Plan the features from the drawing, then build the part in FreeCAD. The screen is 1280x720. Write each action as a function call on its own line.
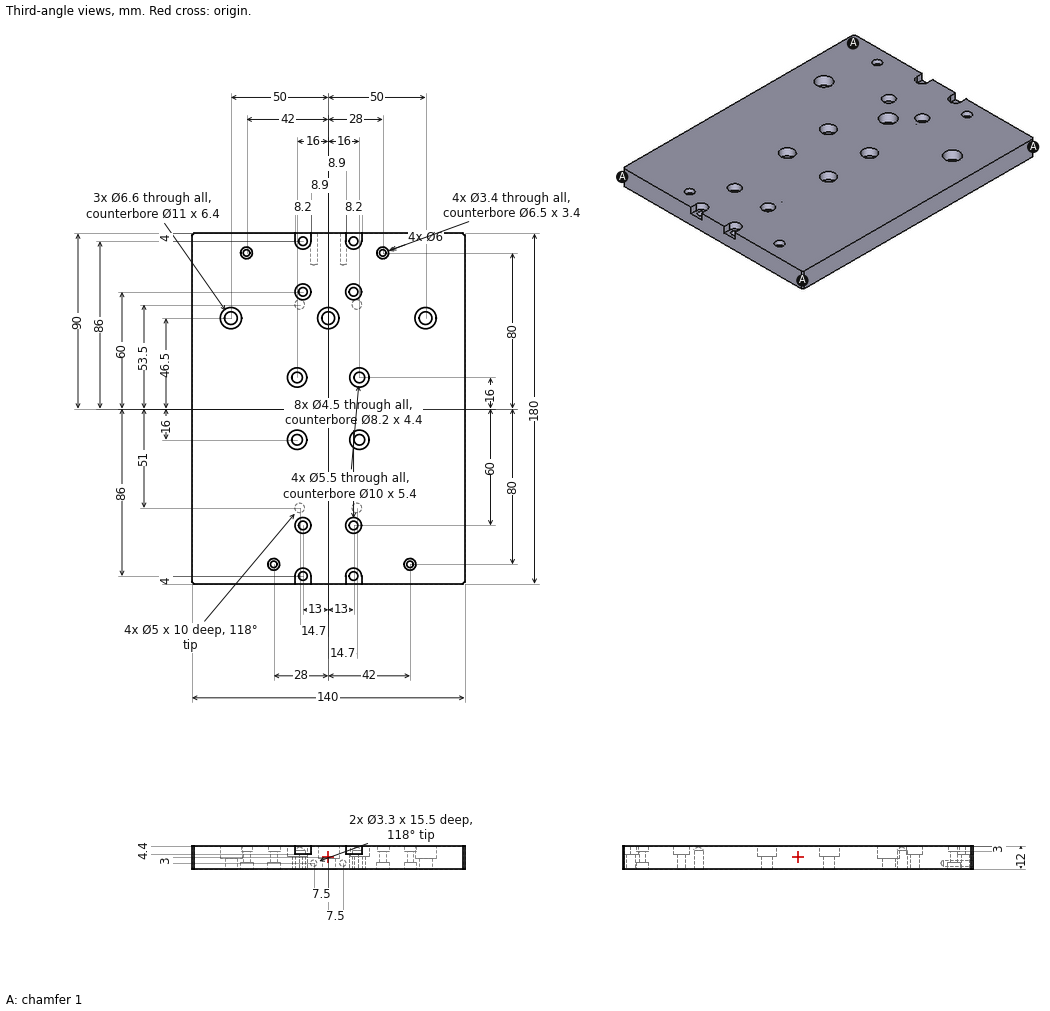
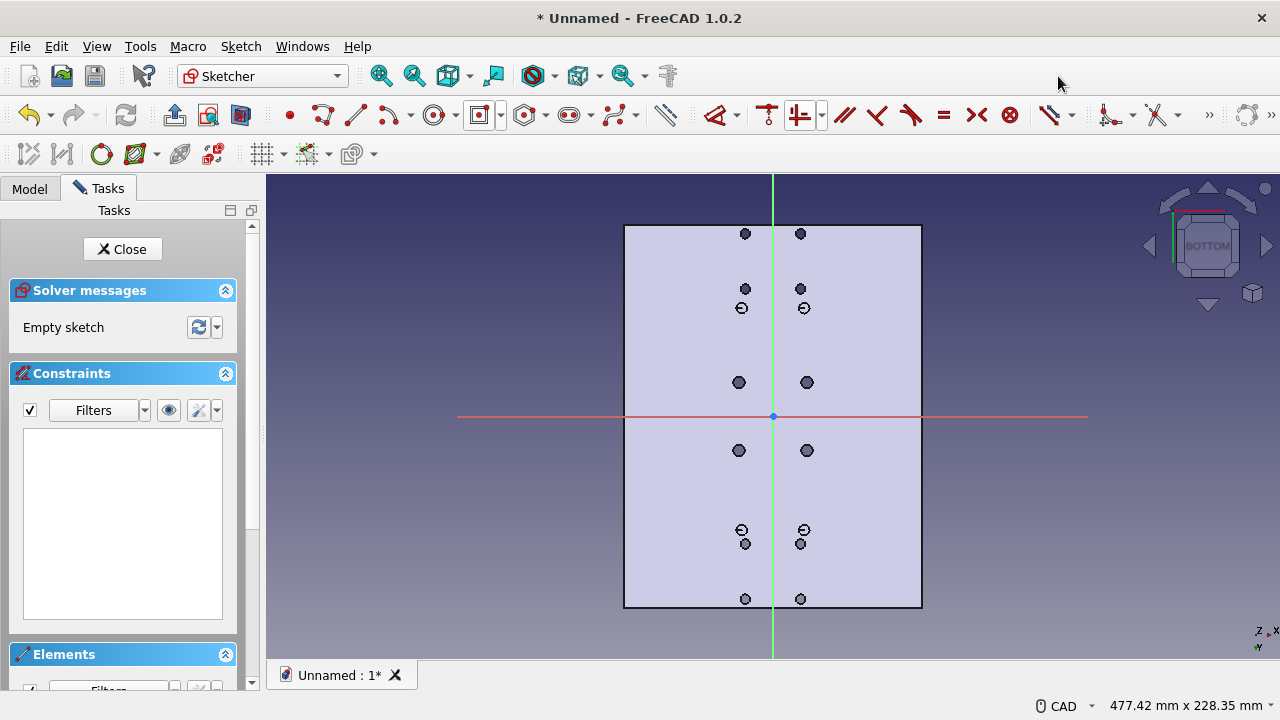
click(434, 116)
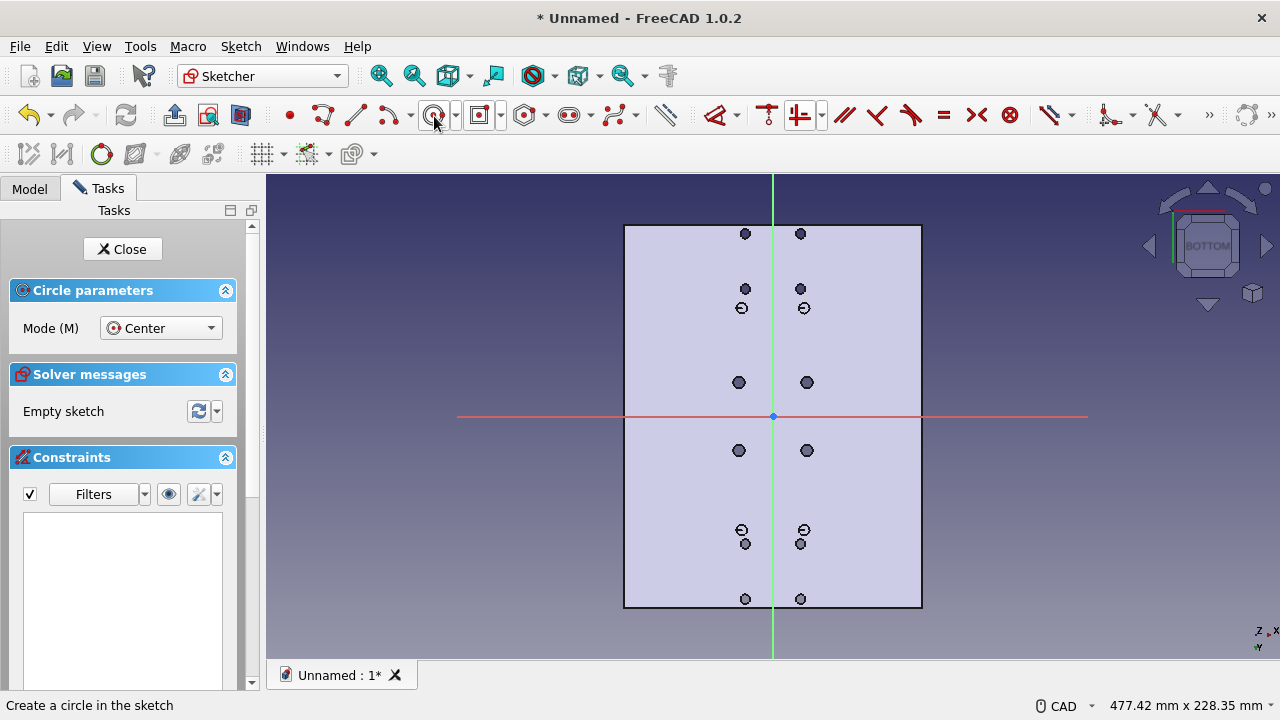
scroll(832, 586, up, 10)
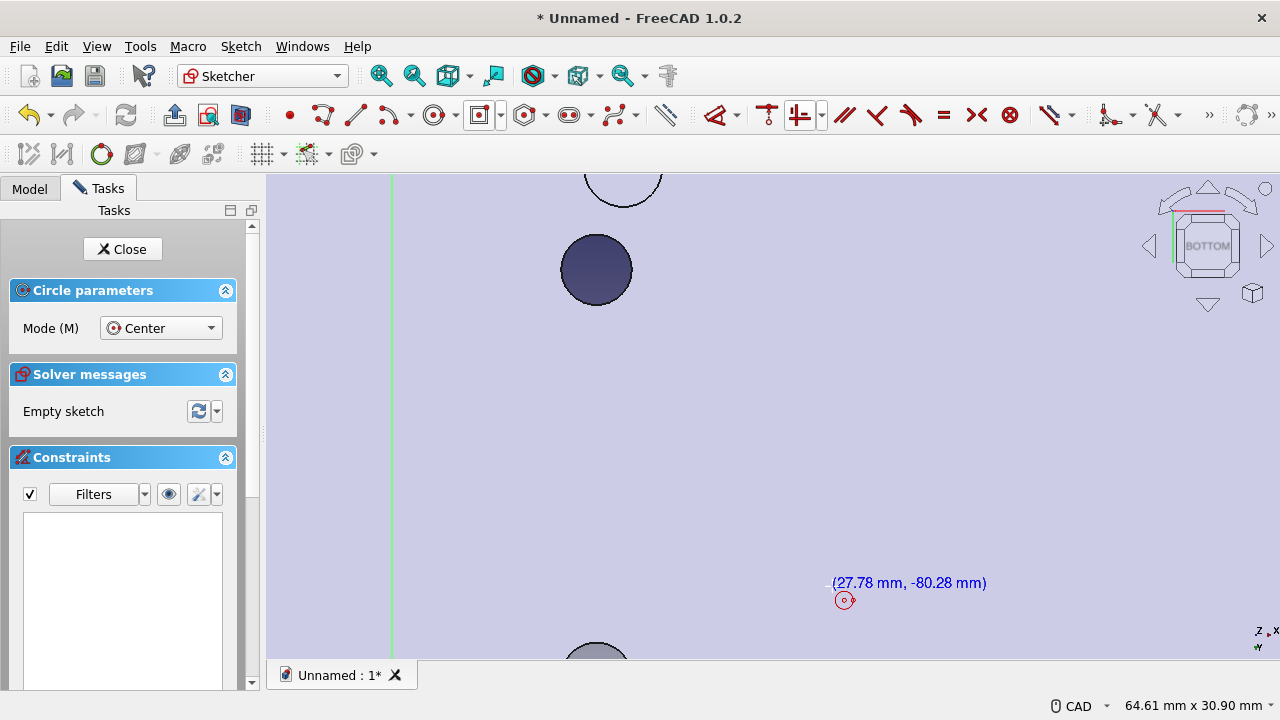
scroll(743, 552, down, 11)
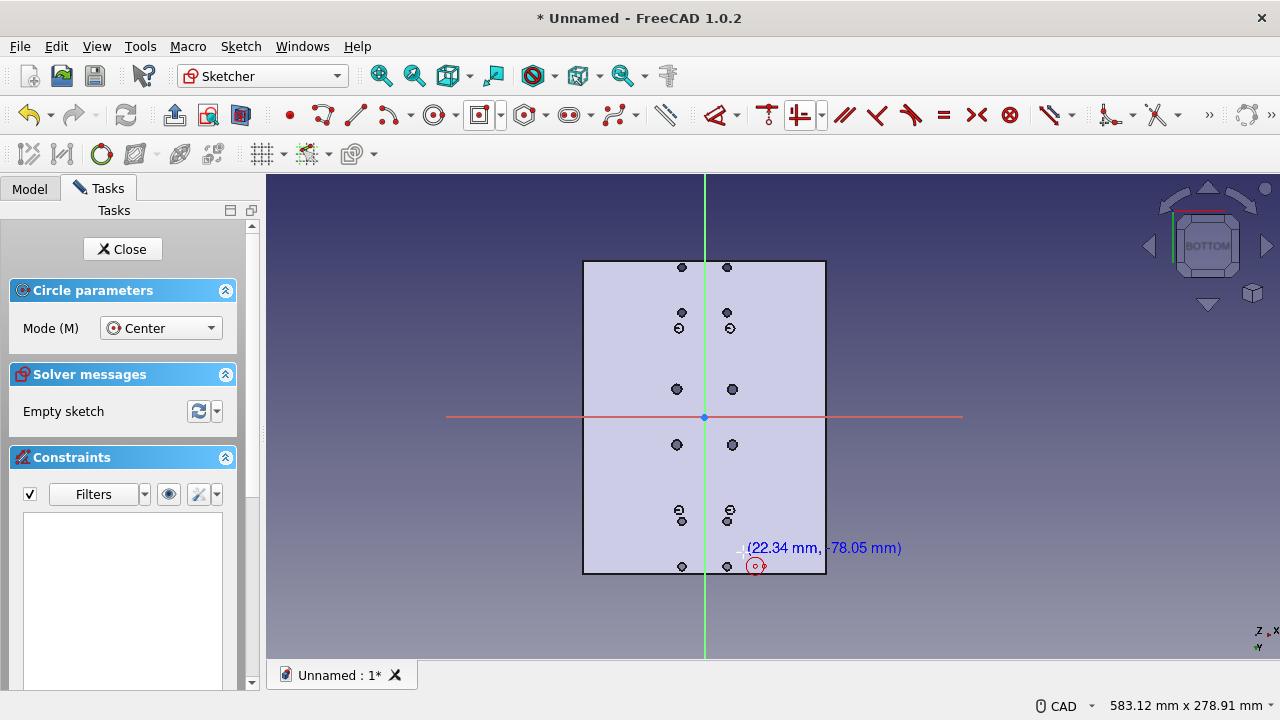
click(753, 556)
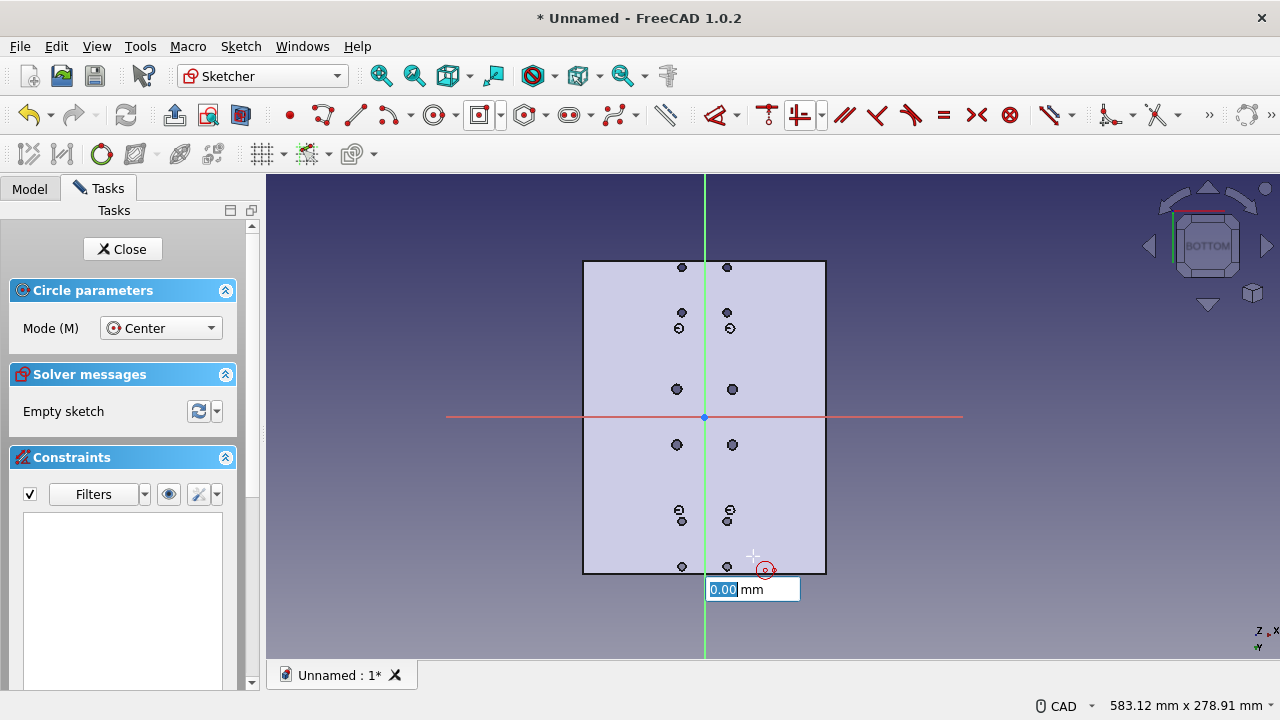
scroll(755, 554, up, 9)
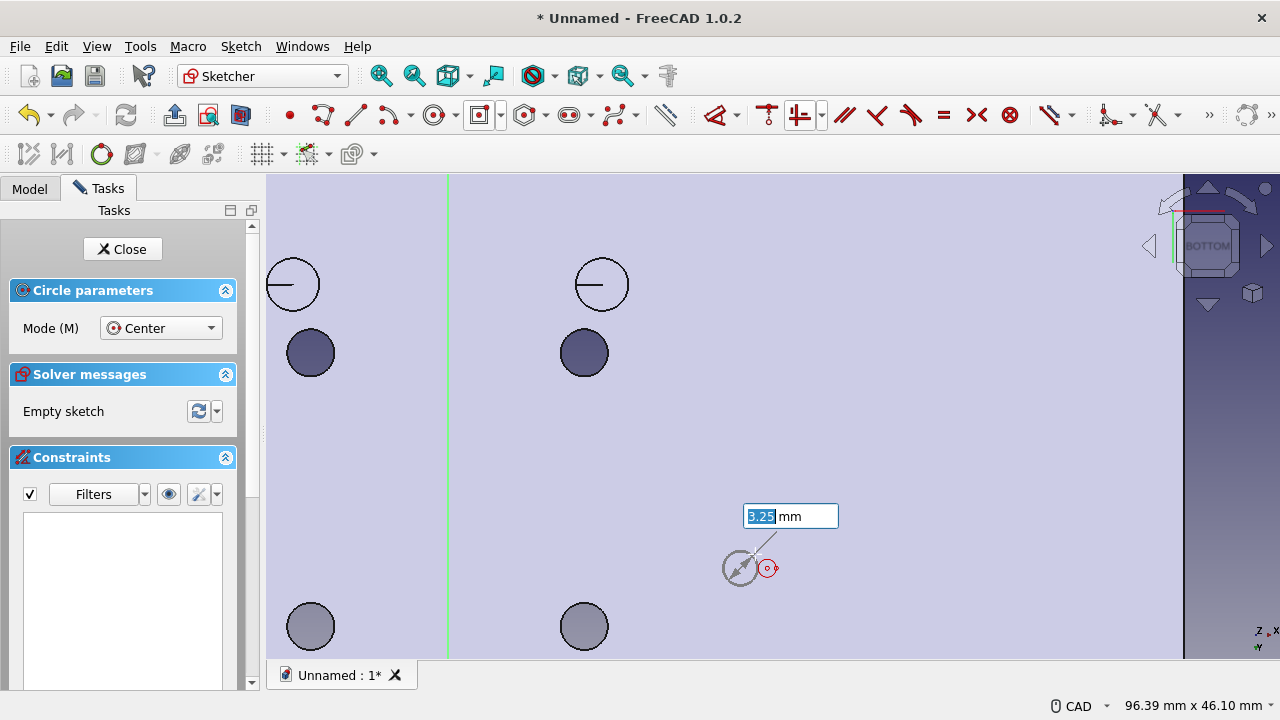
click(755, 551)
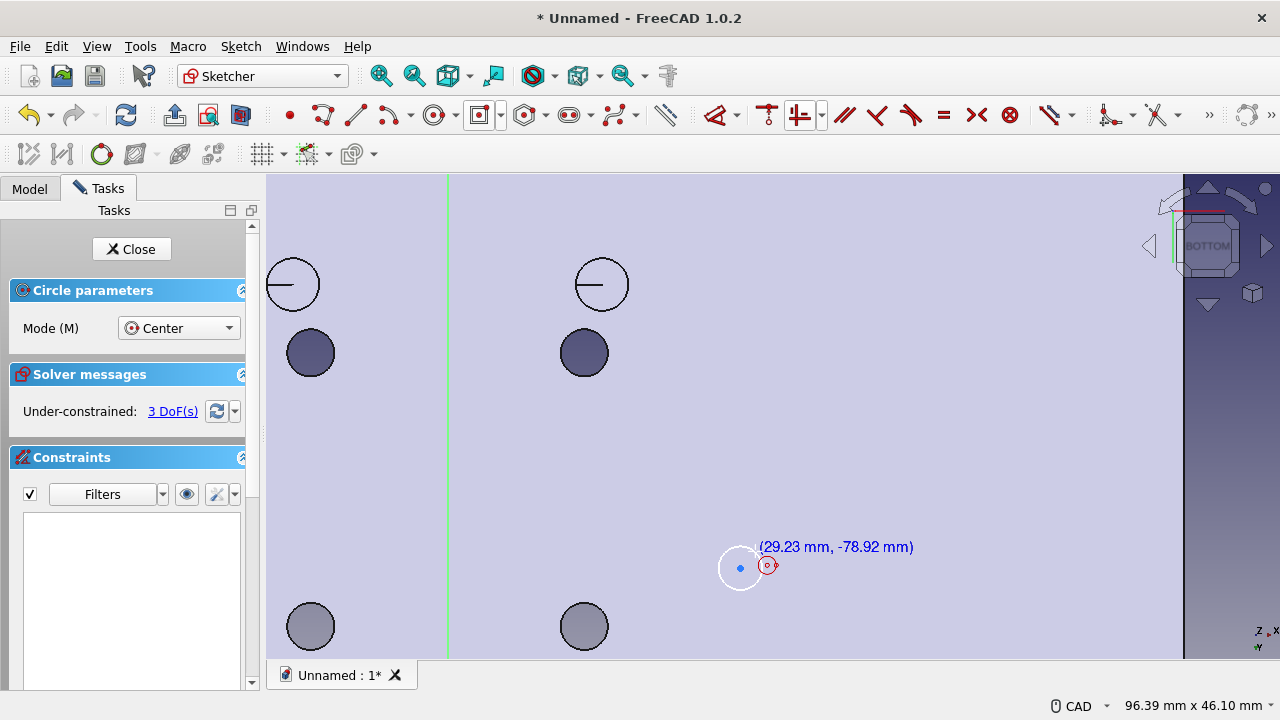
scroll(755, 554, down, 9)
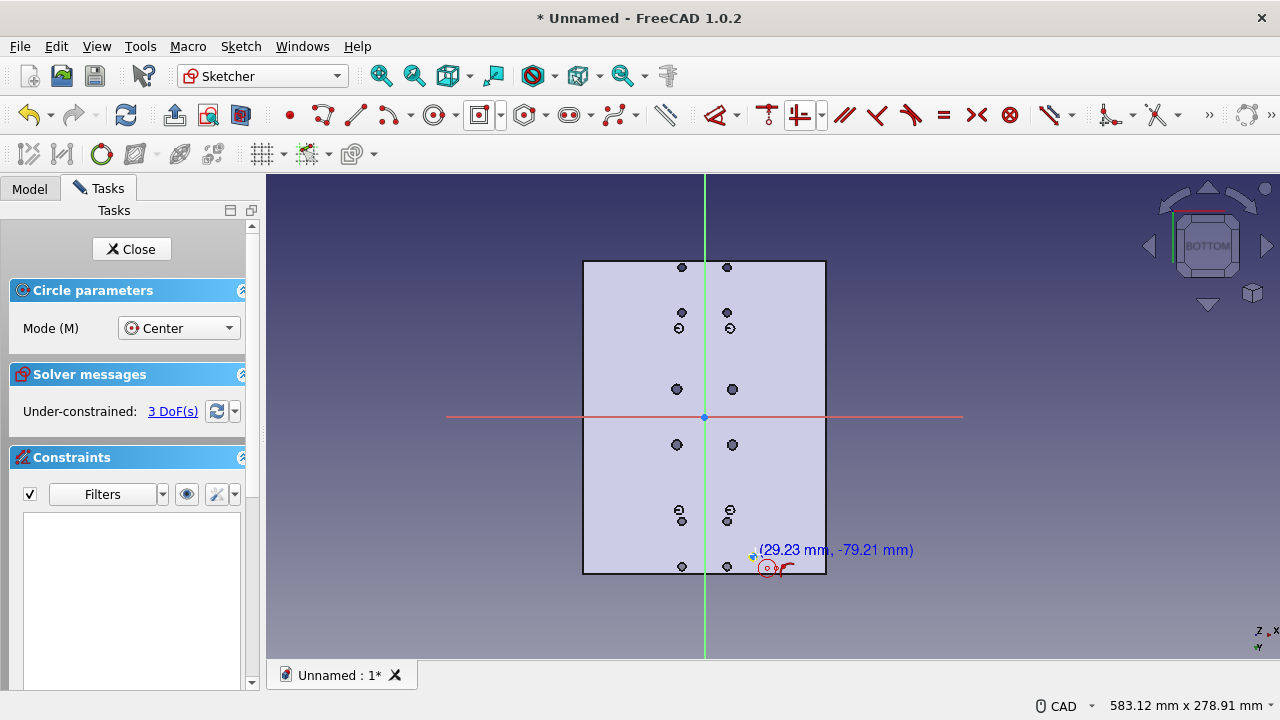
scroll(632, 556, up, 11)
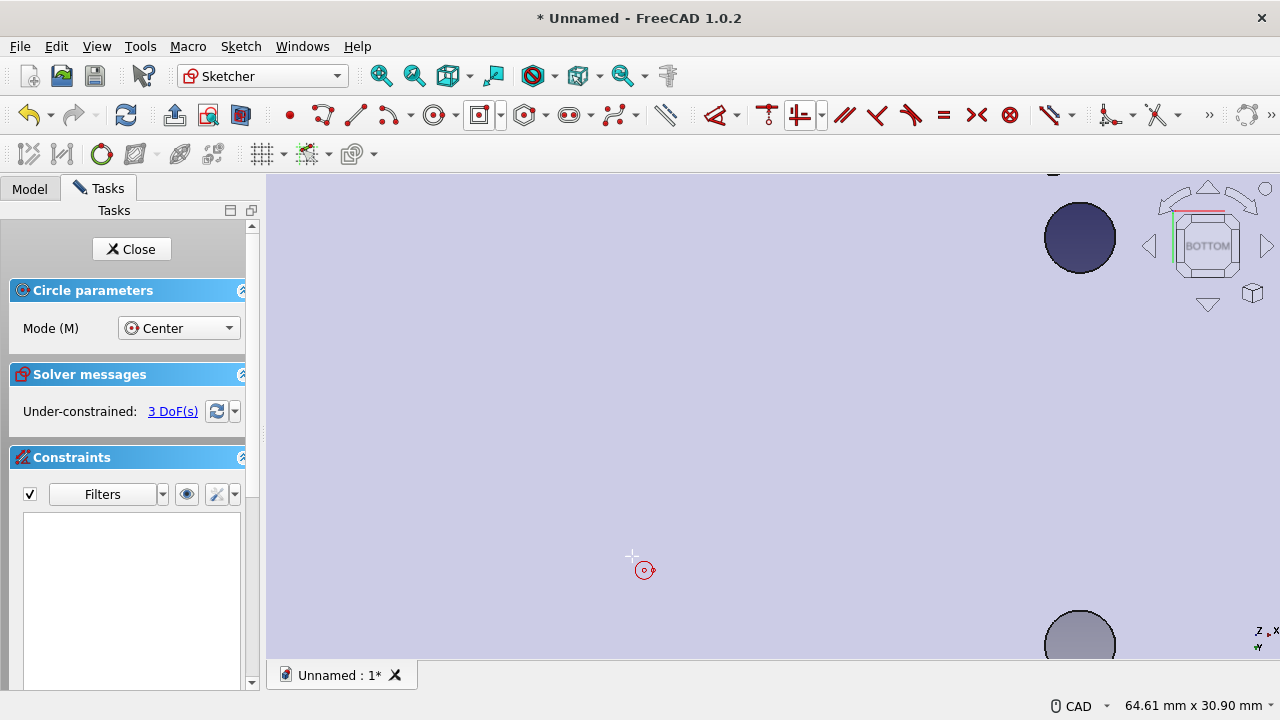
scroll(632, 556, down, 11)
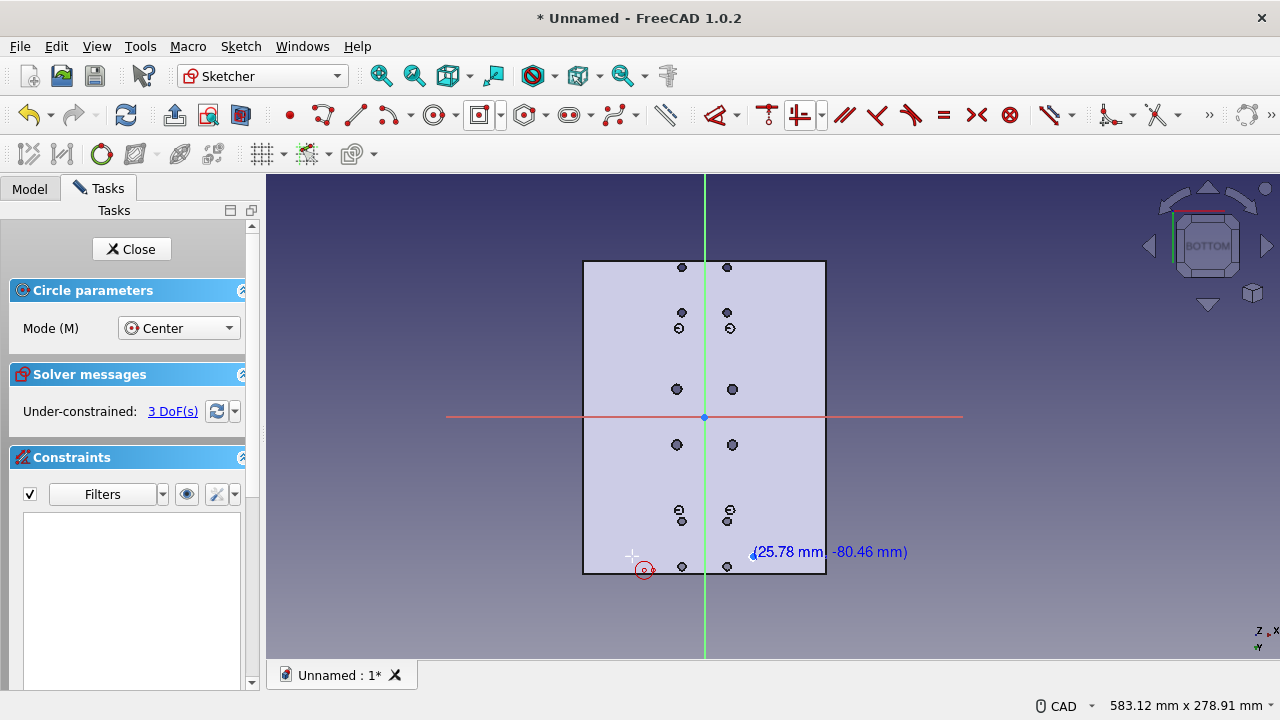
click(632, 556)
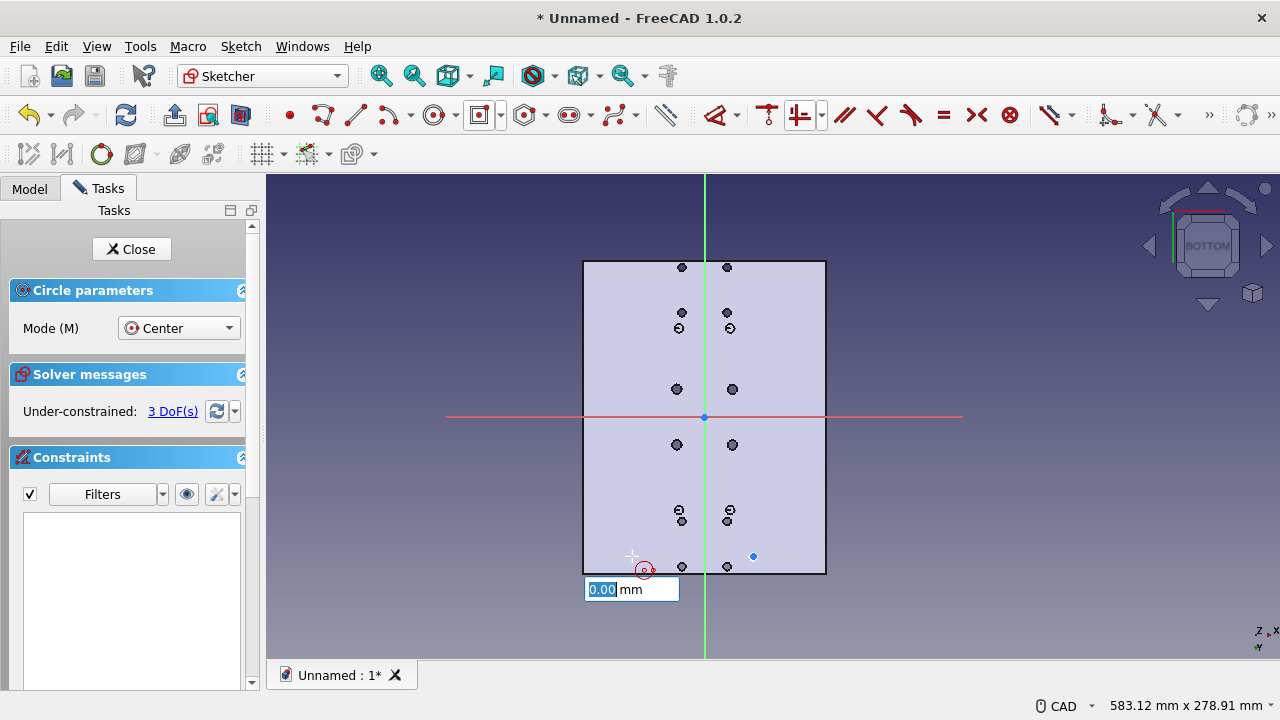
scroll(634, 554, up, 9)